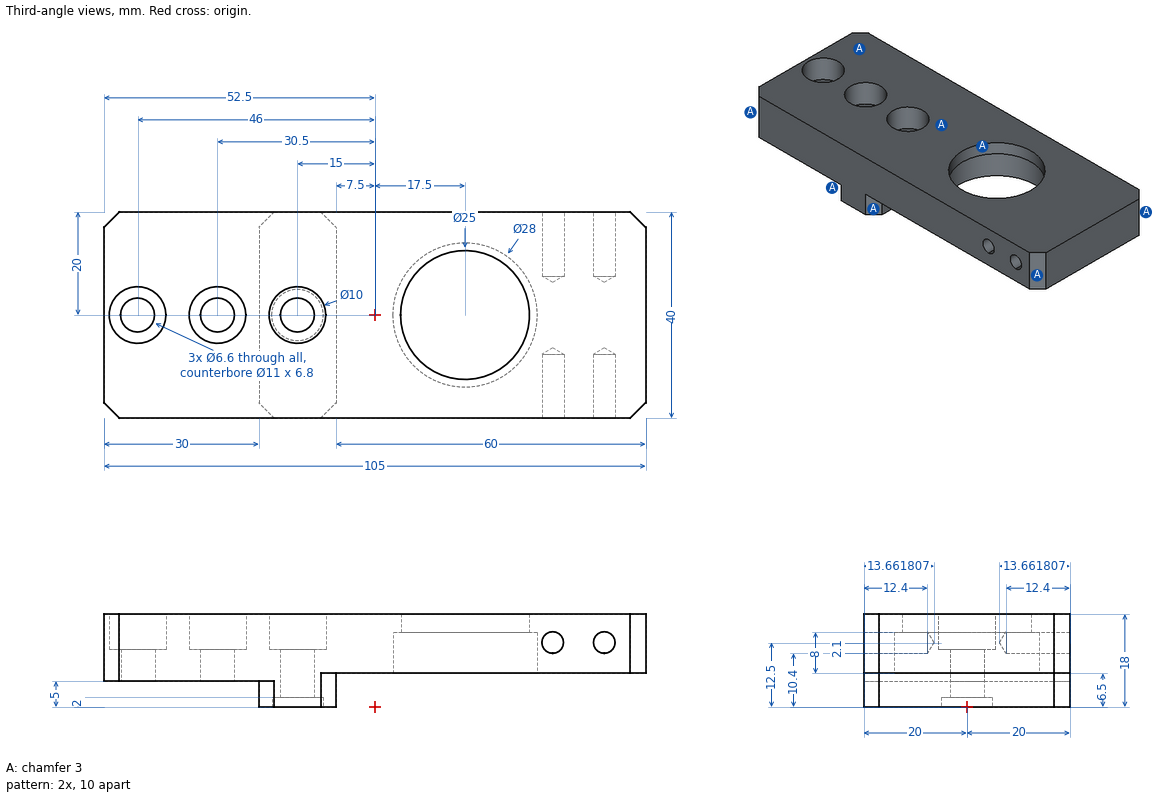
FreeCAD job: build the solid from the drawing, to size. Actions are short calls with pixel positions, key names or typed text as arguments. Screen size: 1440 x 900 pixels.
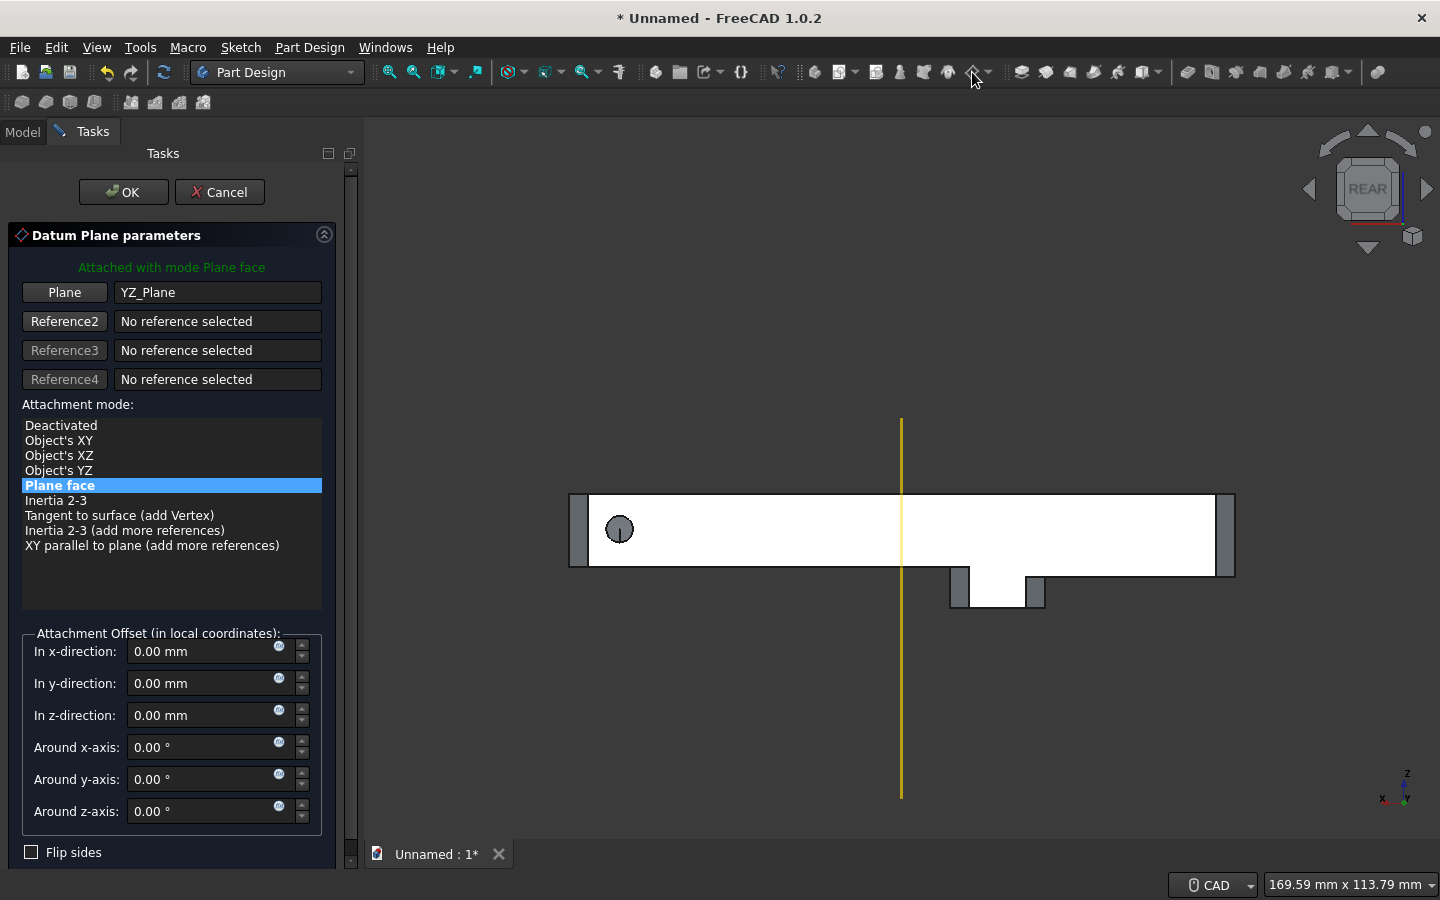
triple_click(210, 715)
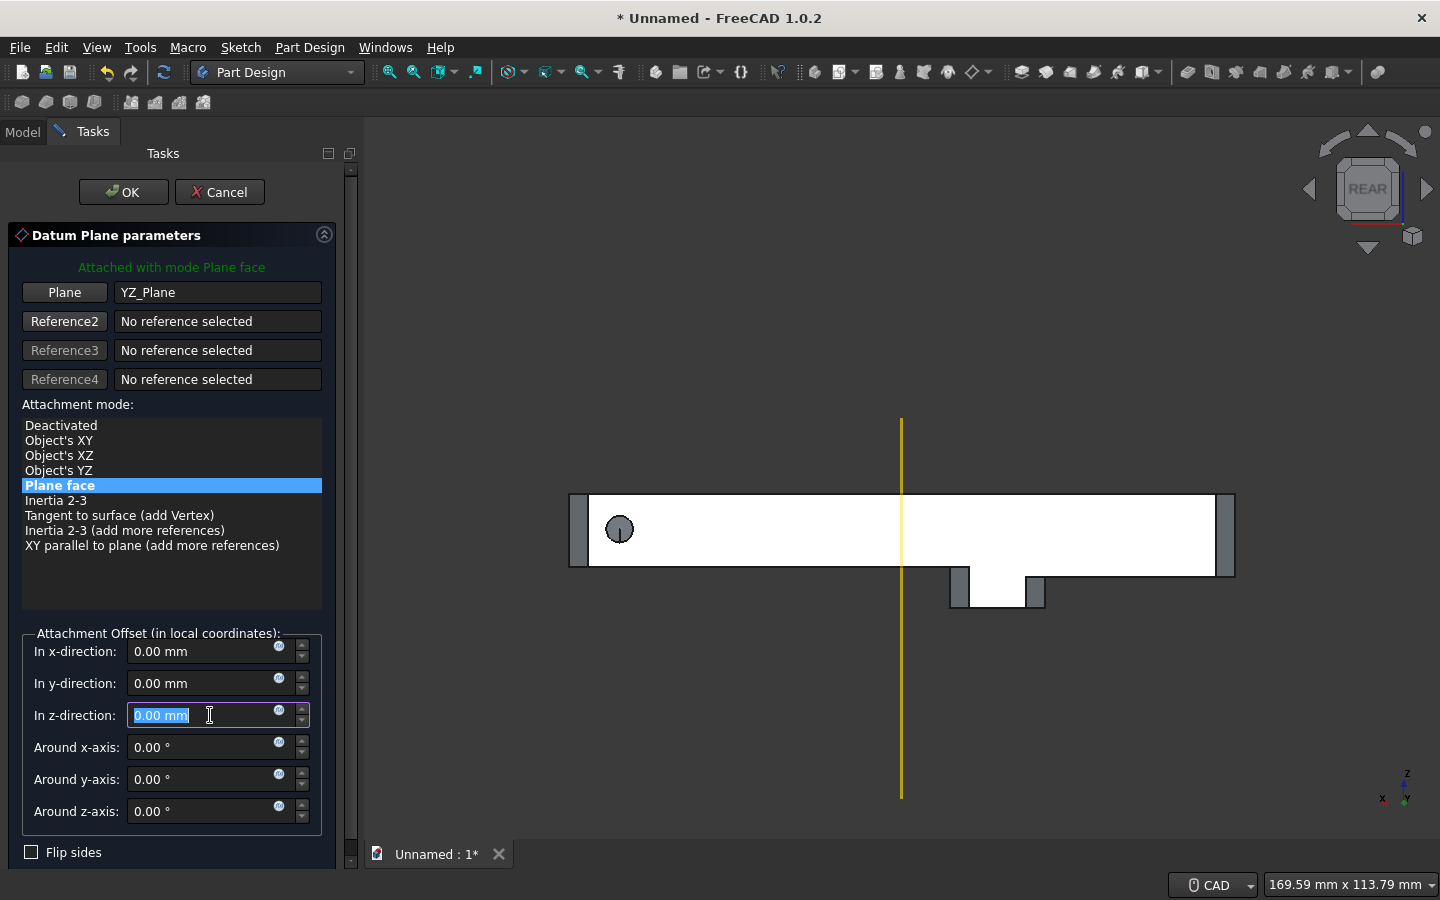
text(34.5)
key(Tab)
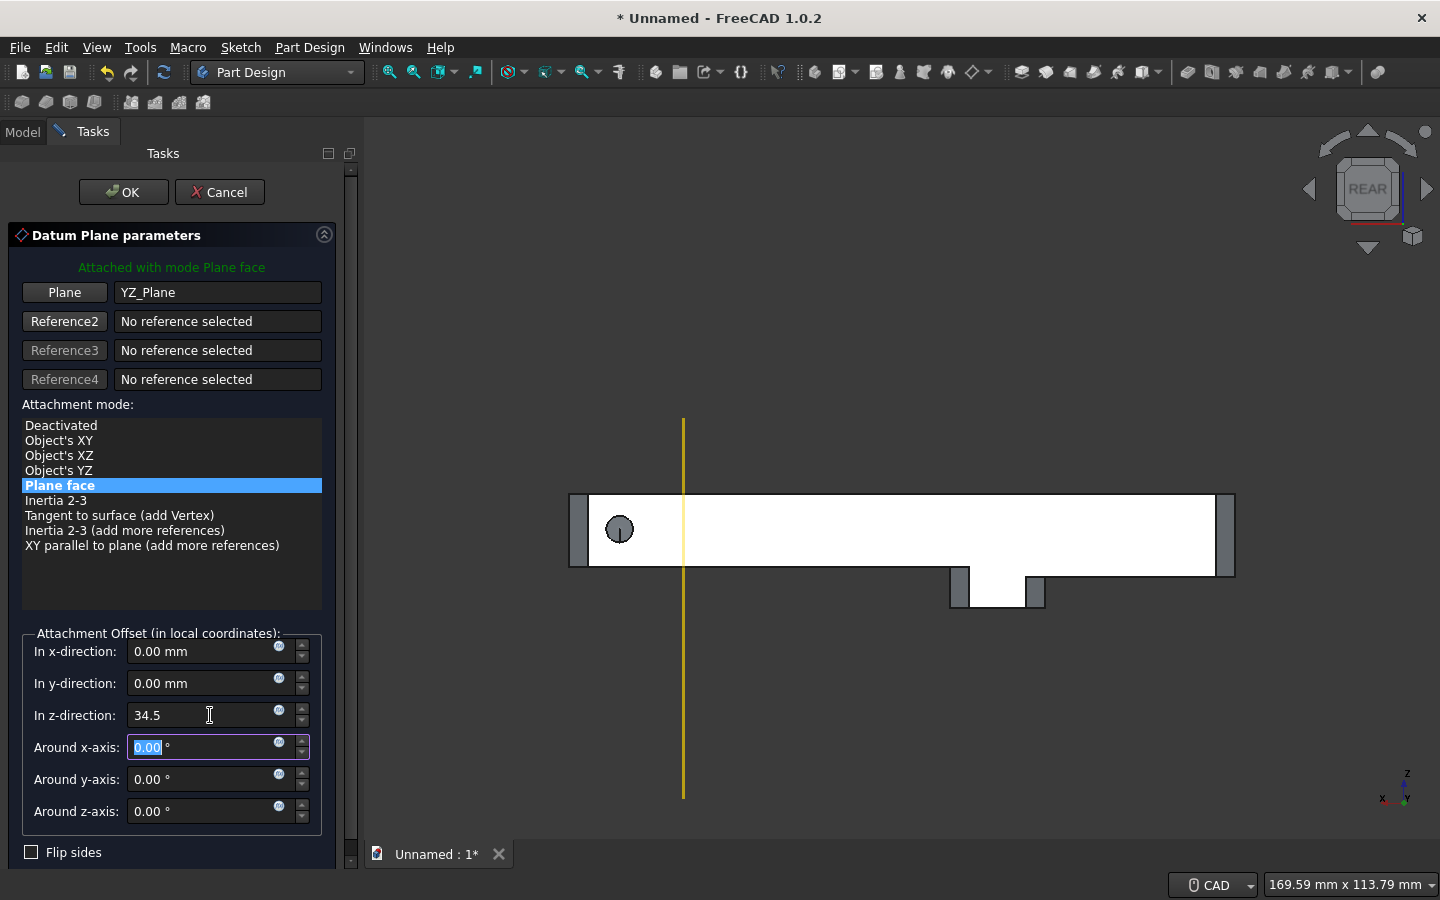
click(124, 192)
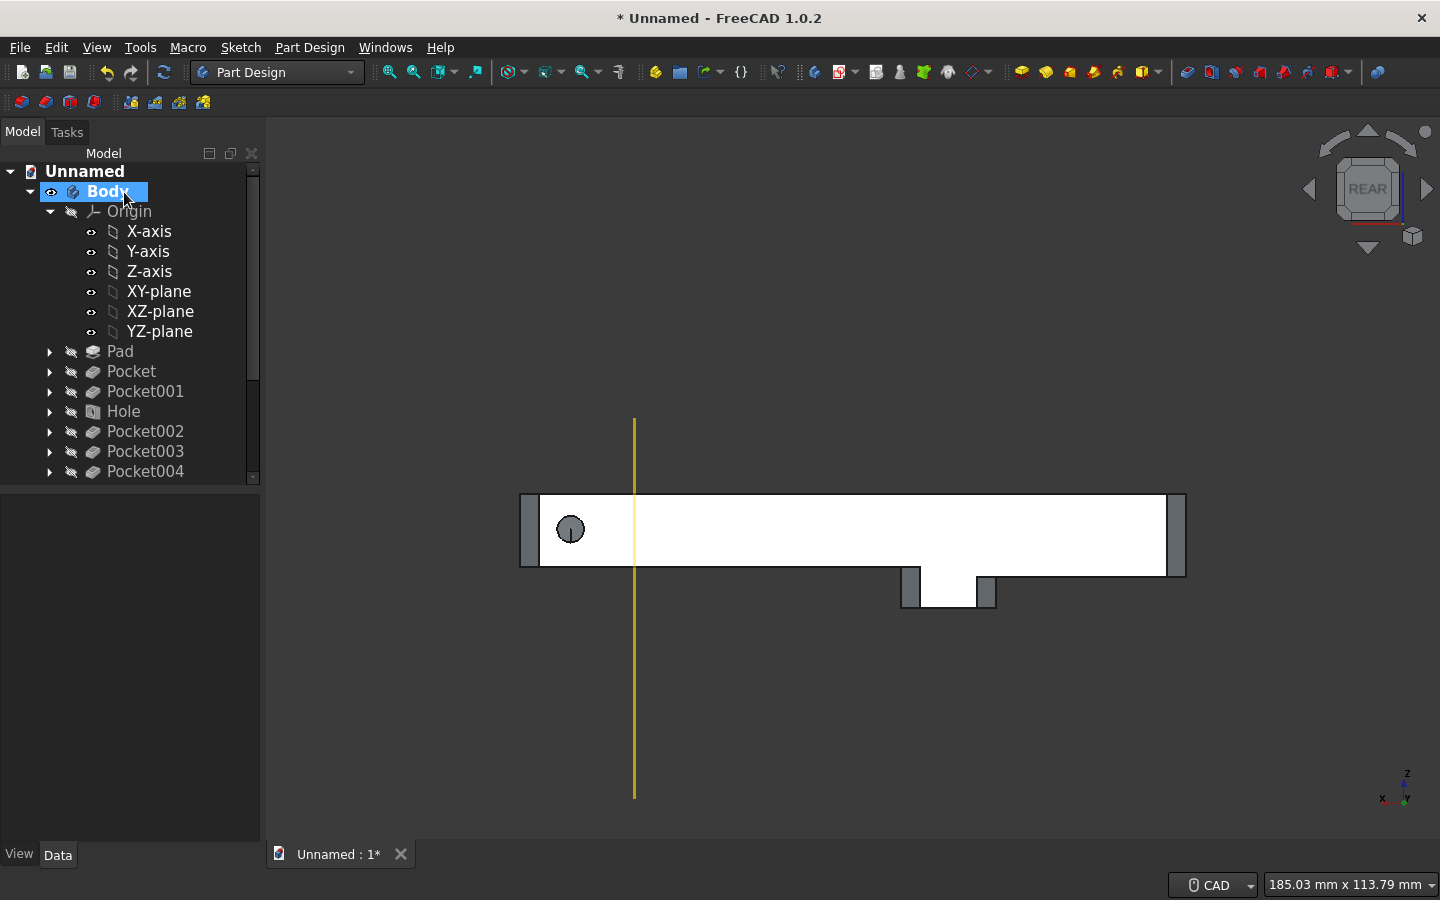
scroll(100, 327, down, 3)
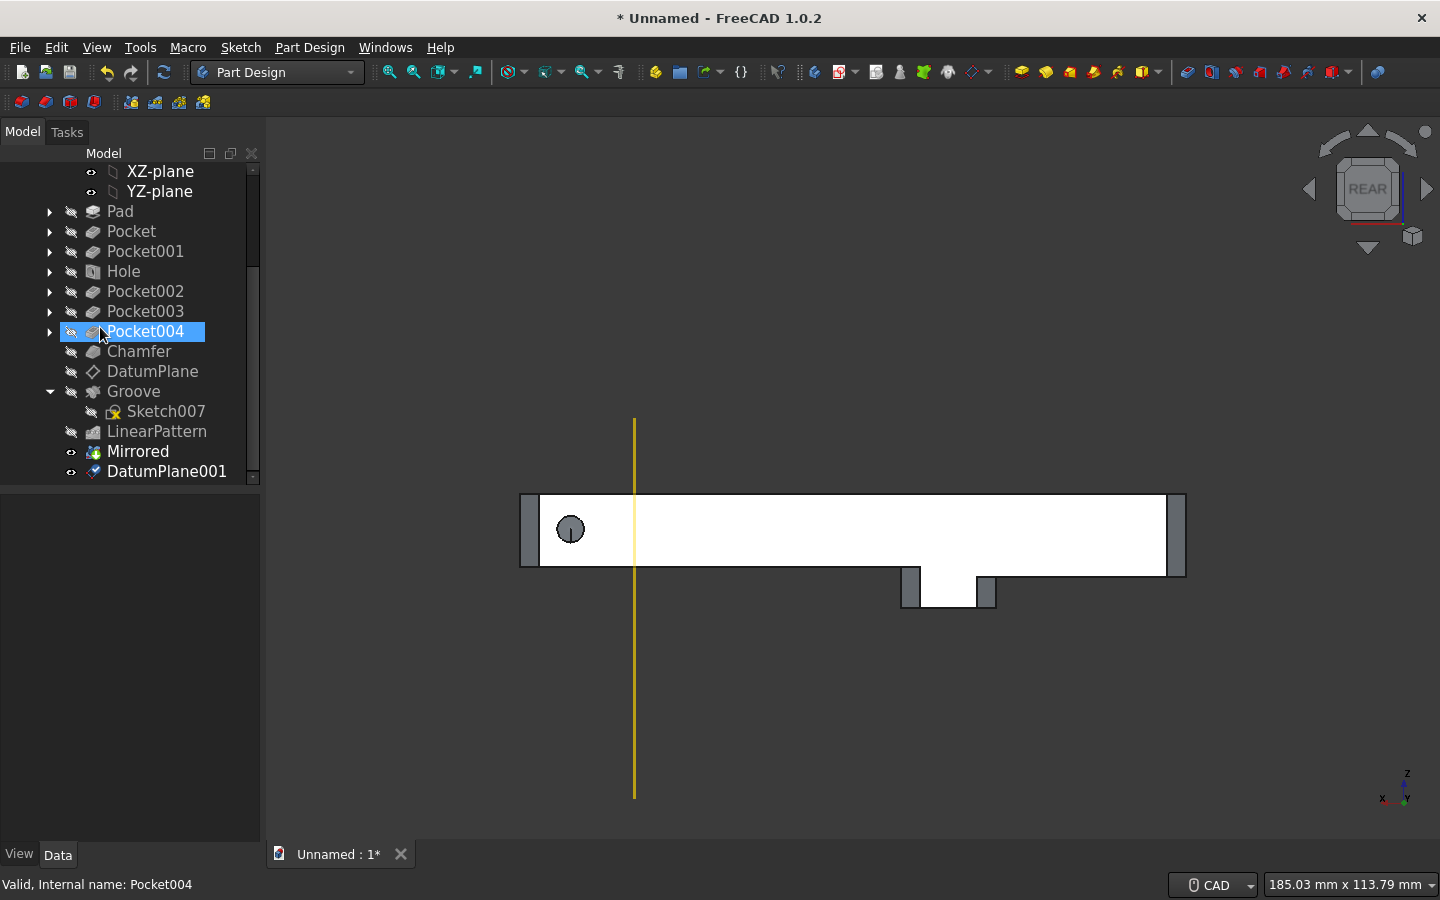
click(116, 472)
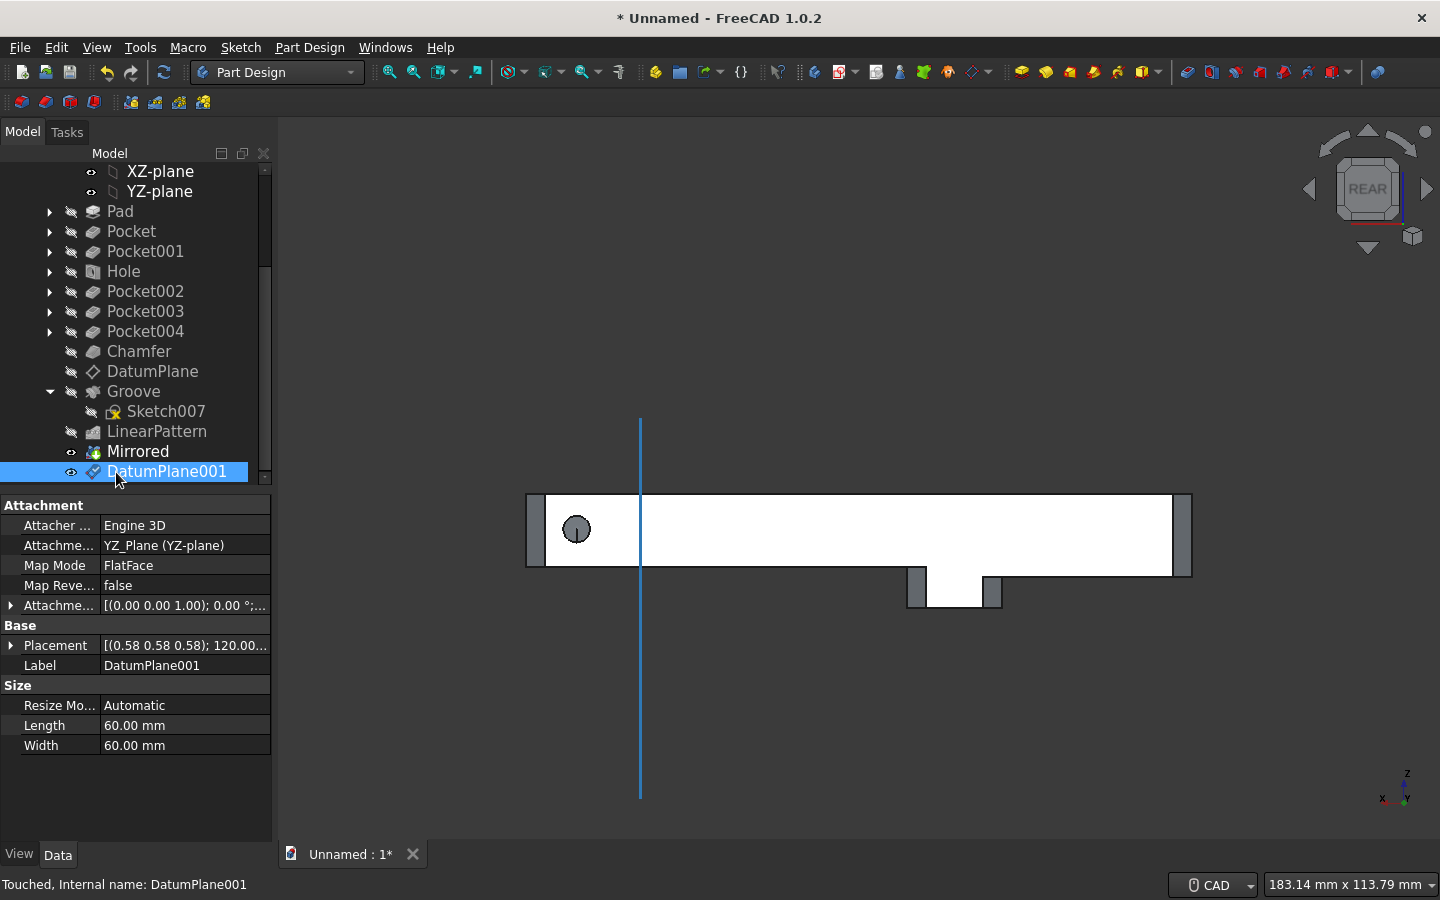
click(840, 72)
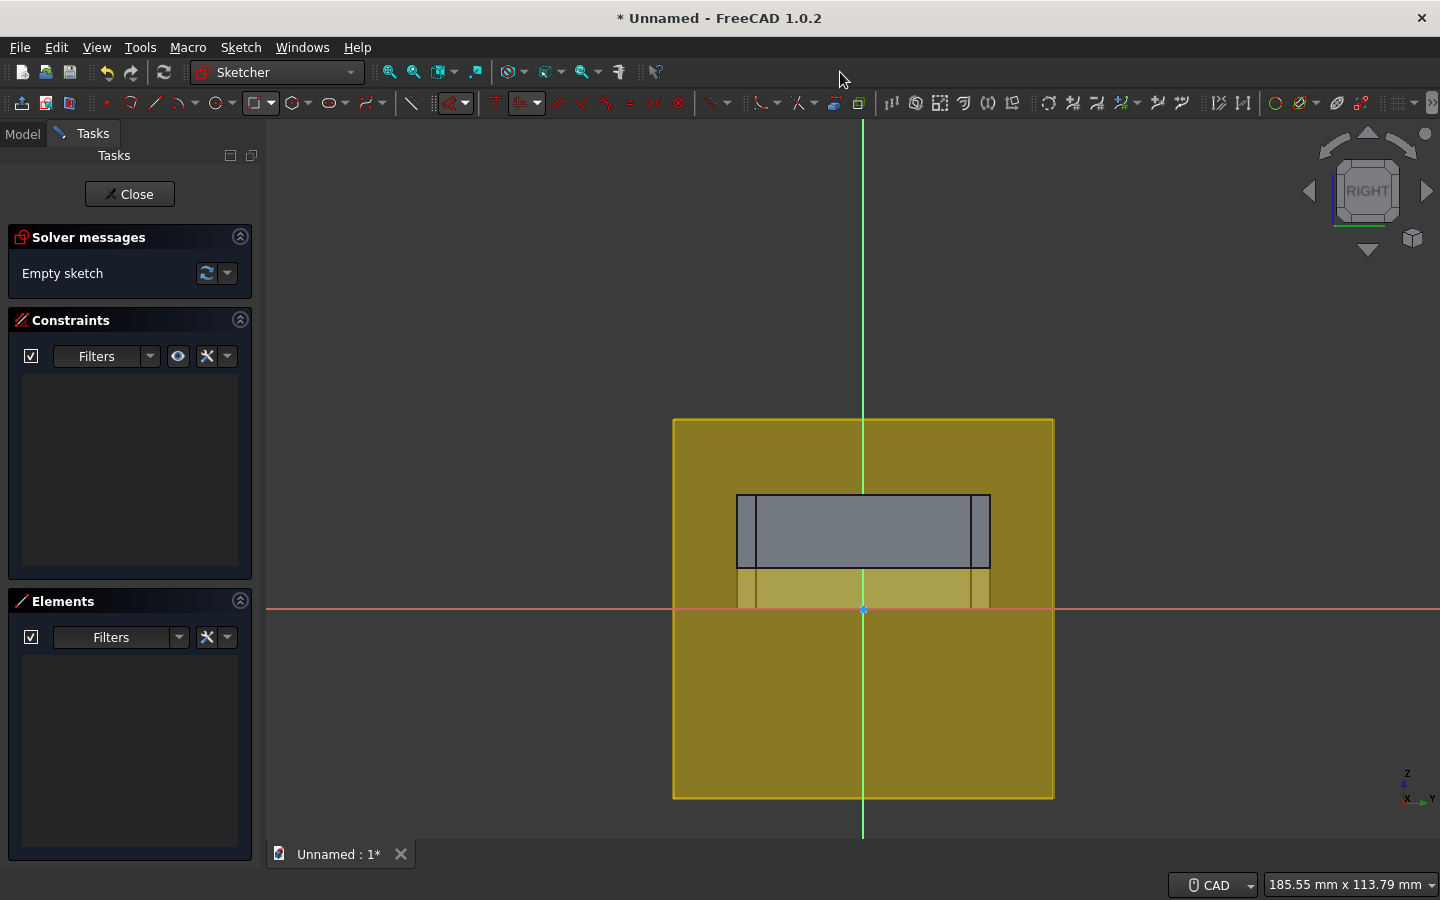
click(70, 104)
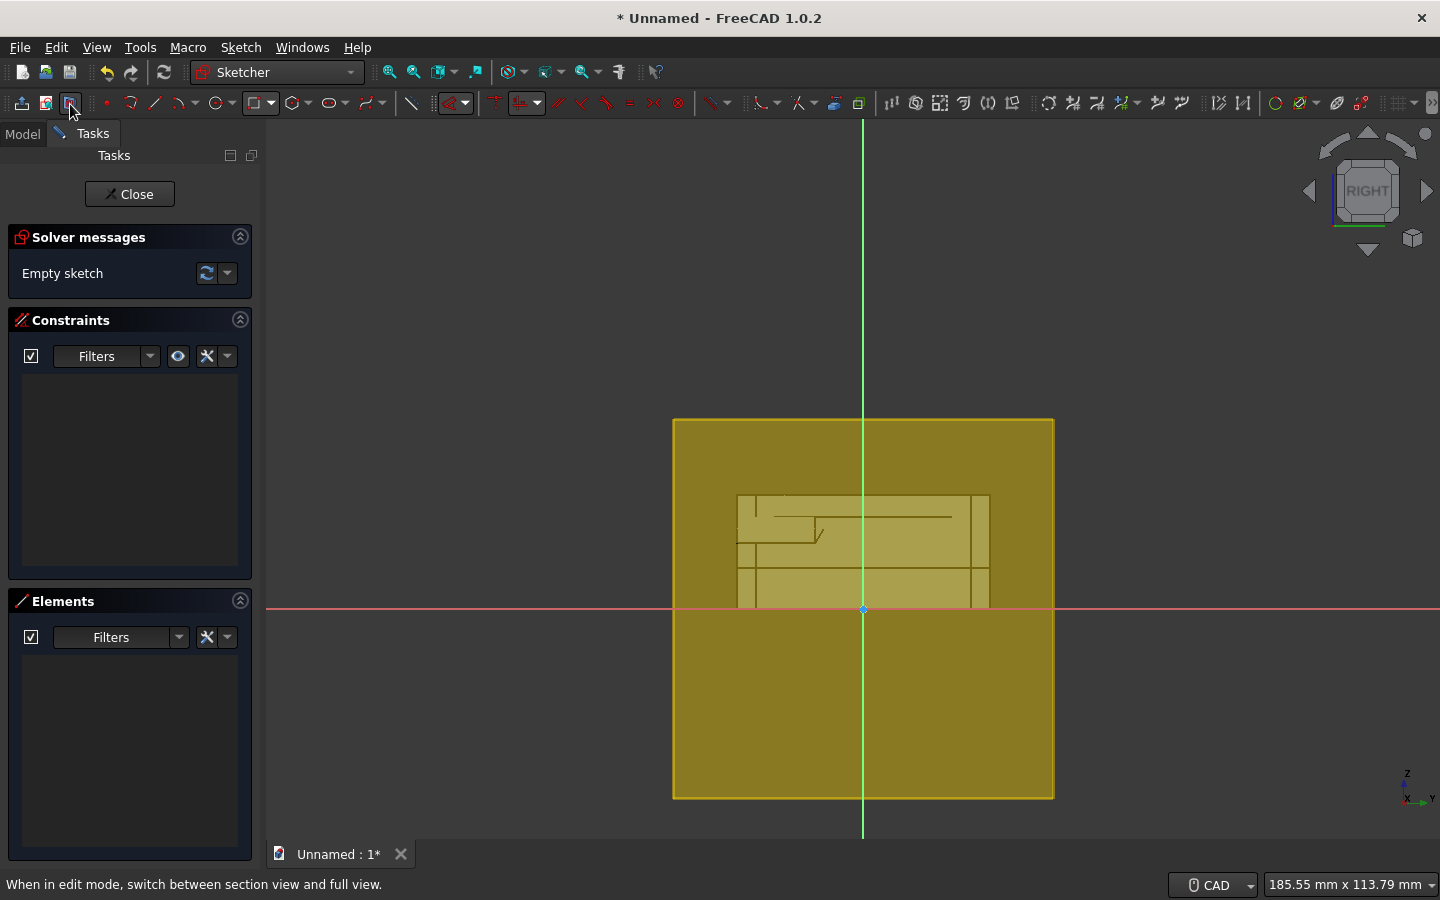
scroll(996, 599, up, 7)